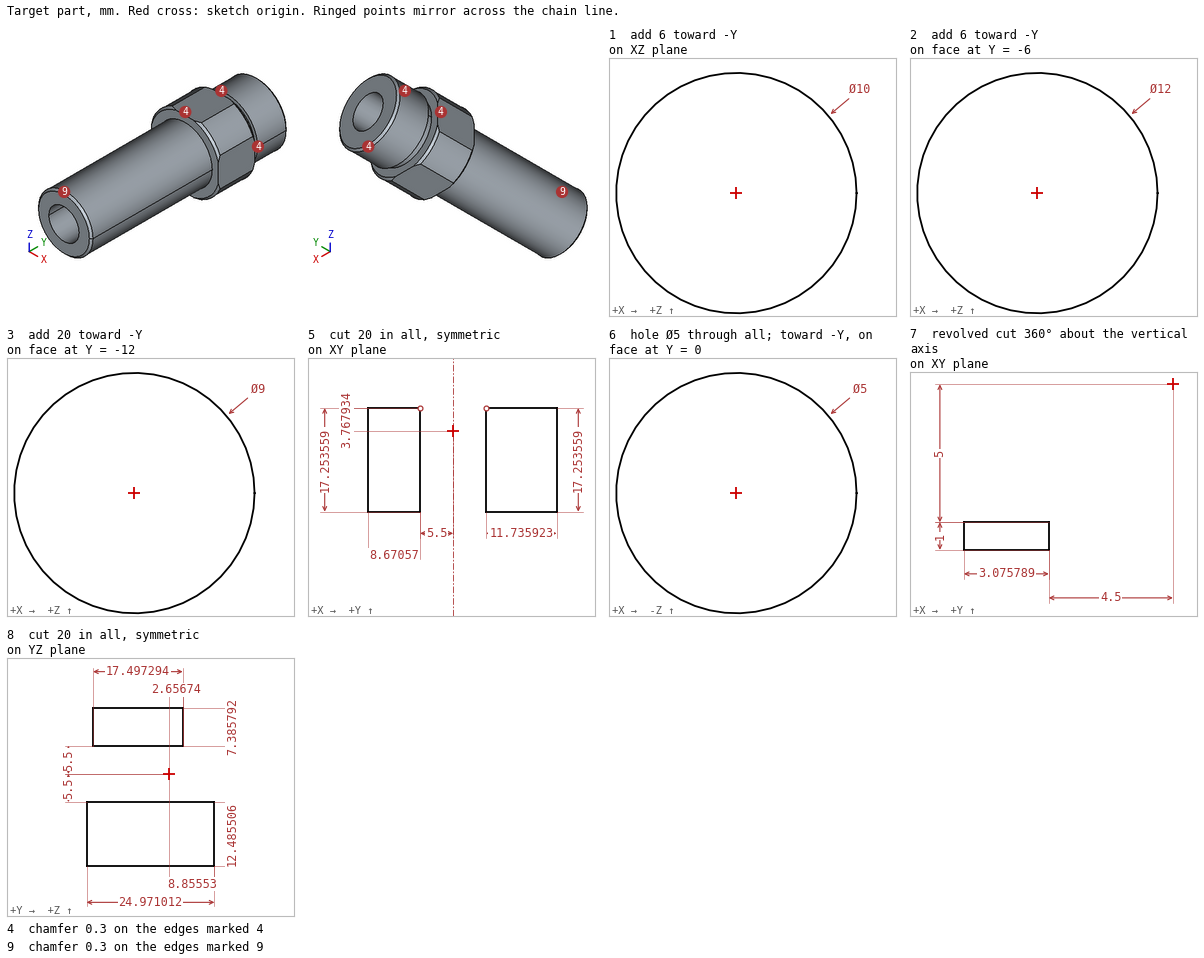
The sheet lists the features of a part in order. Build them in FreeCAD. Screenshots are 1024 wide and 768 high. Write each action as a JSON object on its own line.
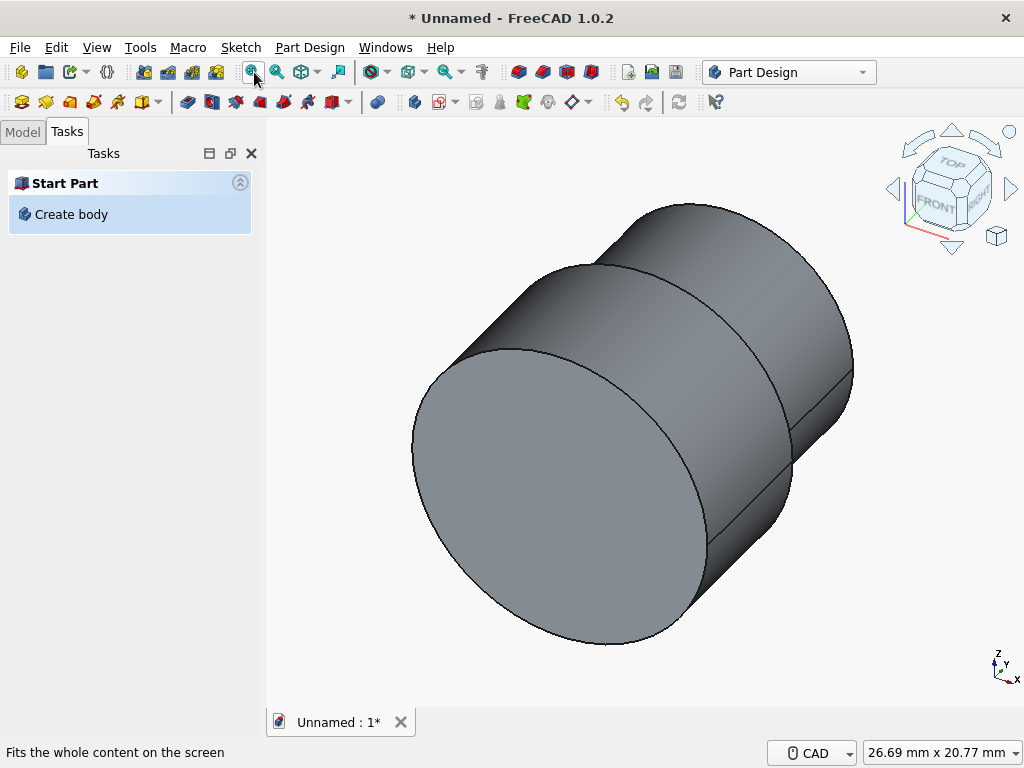
{"action": "left_click", "coordinate": [560, 496]}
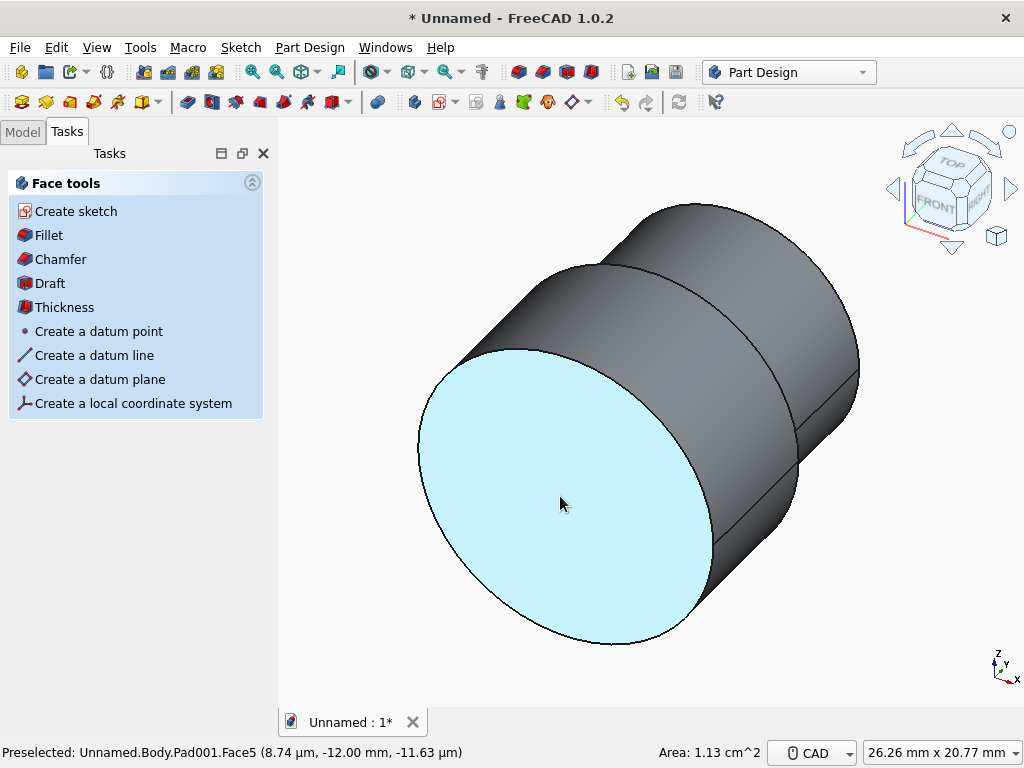
{"action": "left_click", "coordinate": [440, 102]}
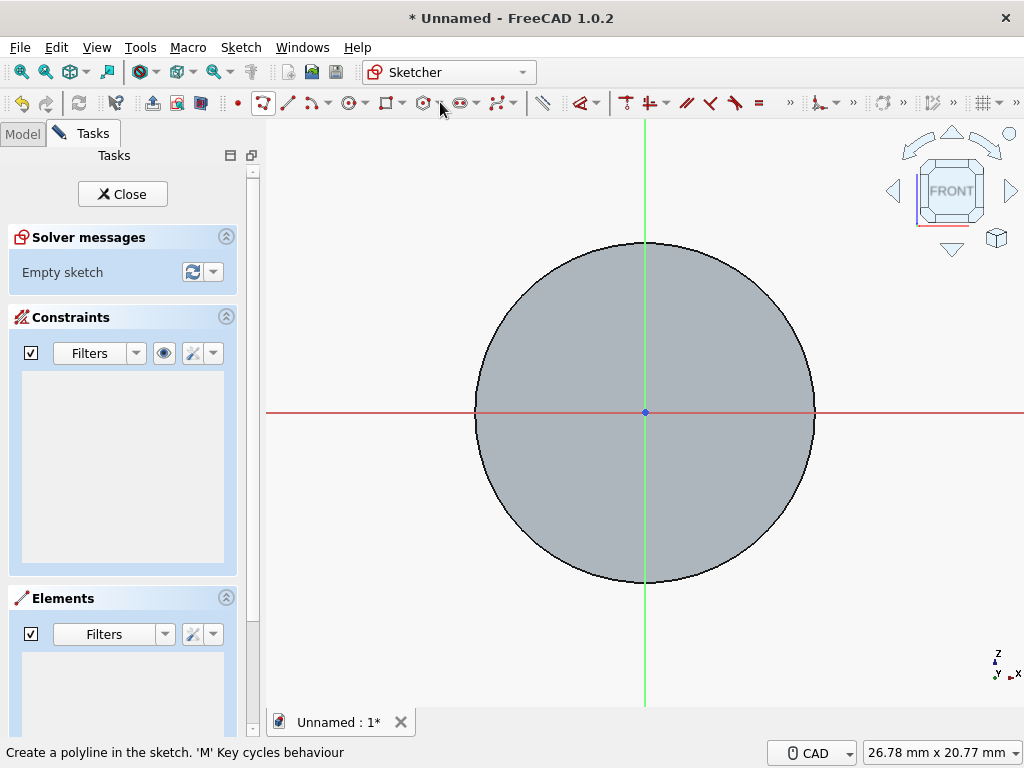
{"action": "scroll", "coordinate": [784, 413], "scroll_direction": "up", "scroll_amount": 2}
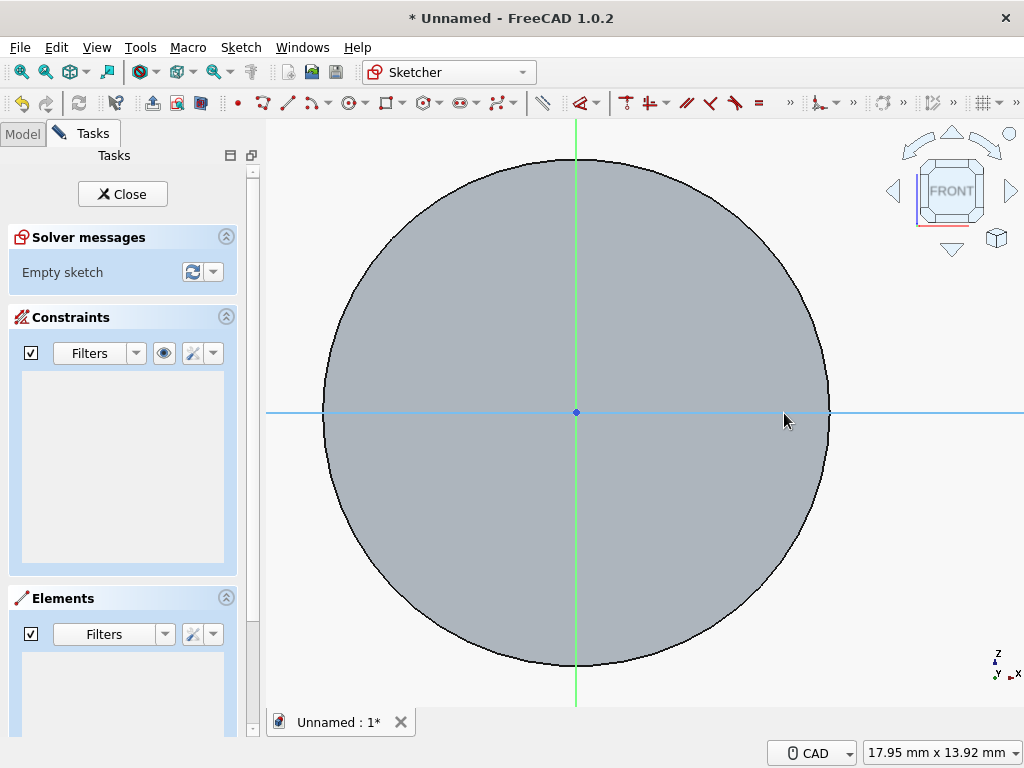
{"action": "key", "text": "g c"}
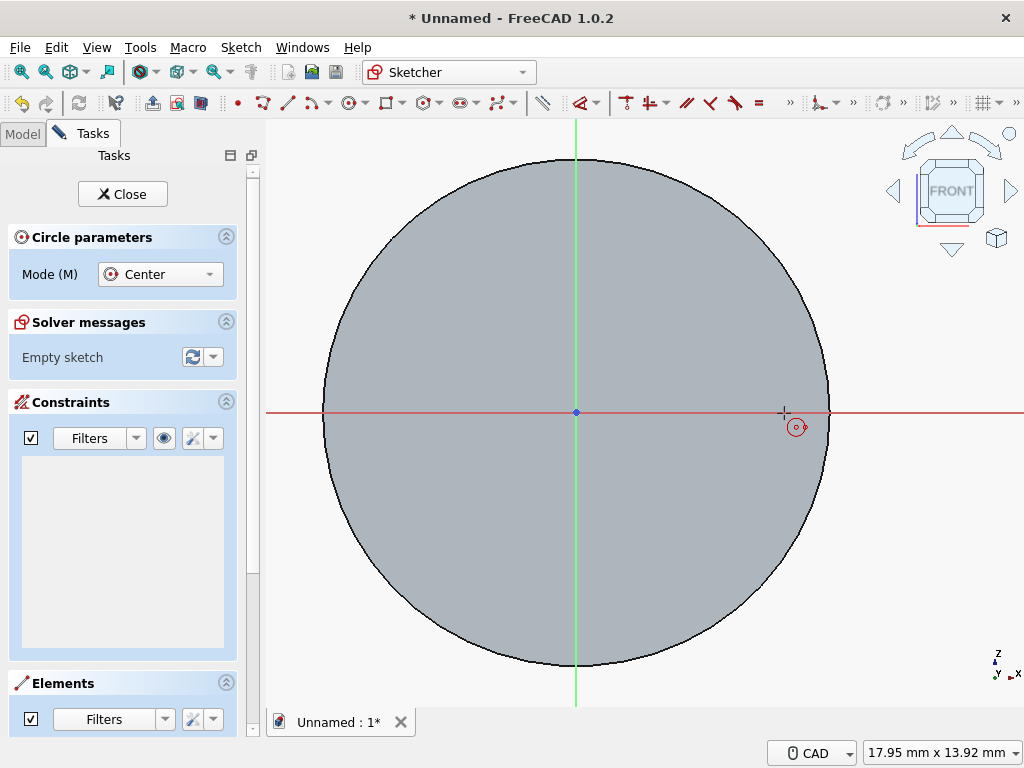
{"action": "left_click", "coordinate": [576, 413]}
{"action": "mouse_move", "coordinate": [711, 278]}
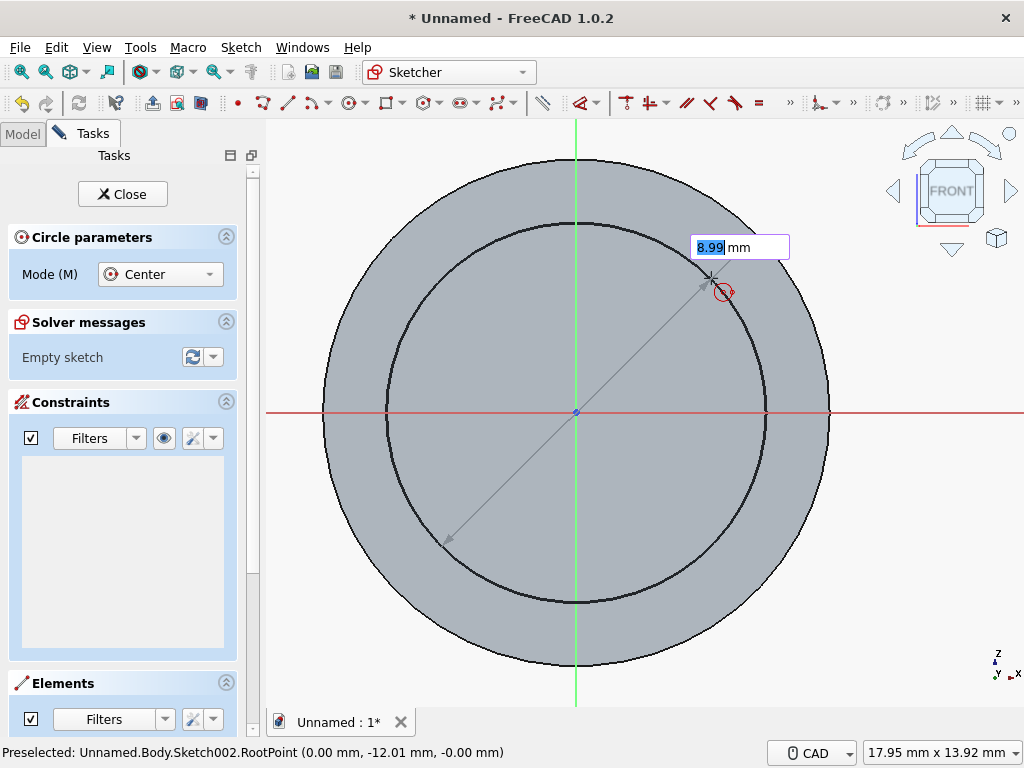
{"action": "type", "text": "9"}
{"action": "key", "text": "Return"}
{"action": "key", "text": "Escape"}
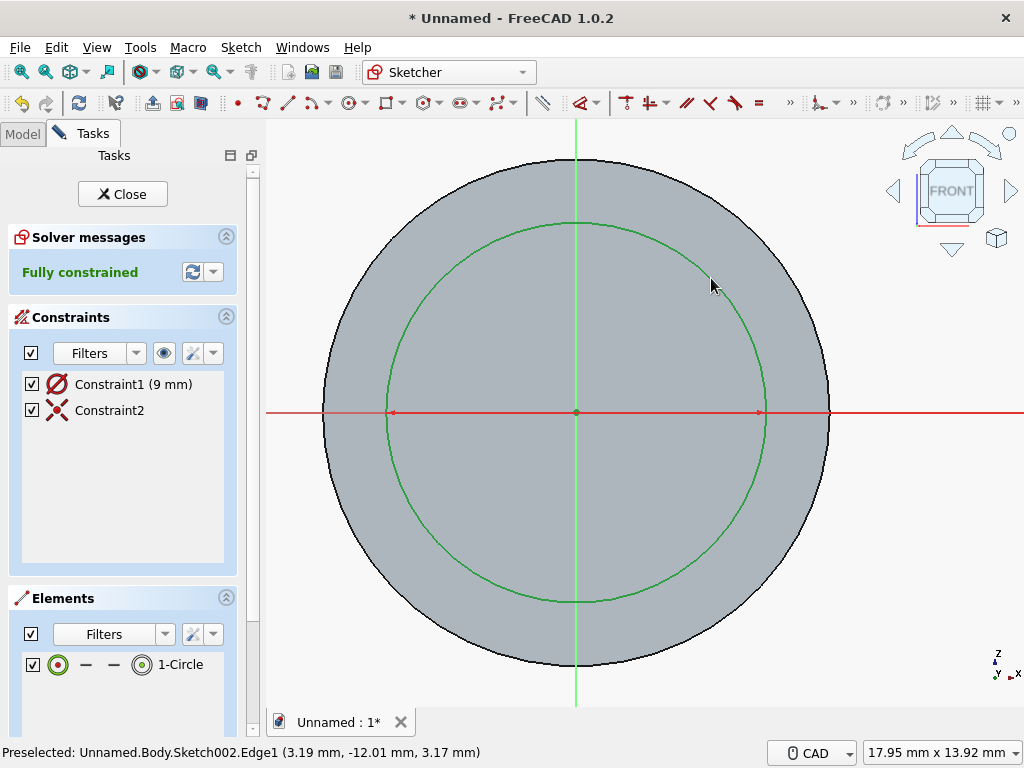
{"action": "left_click", "coordinate": [123, 194]}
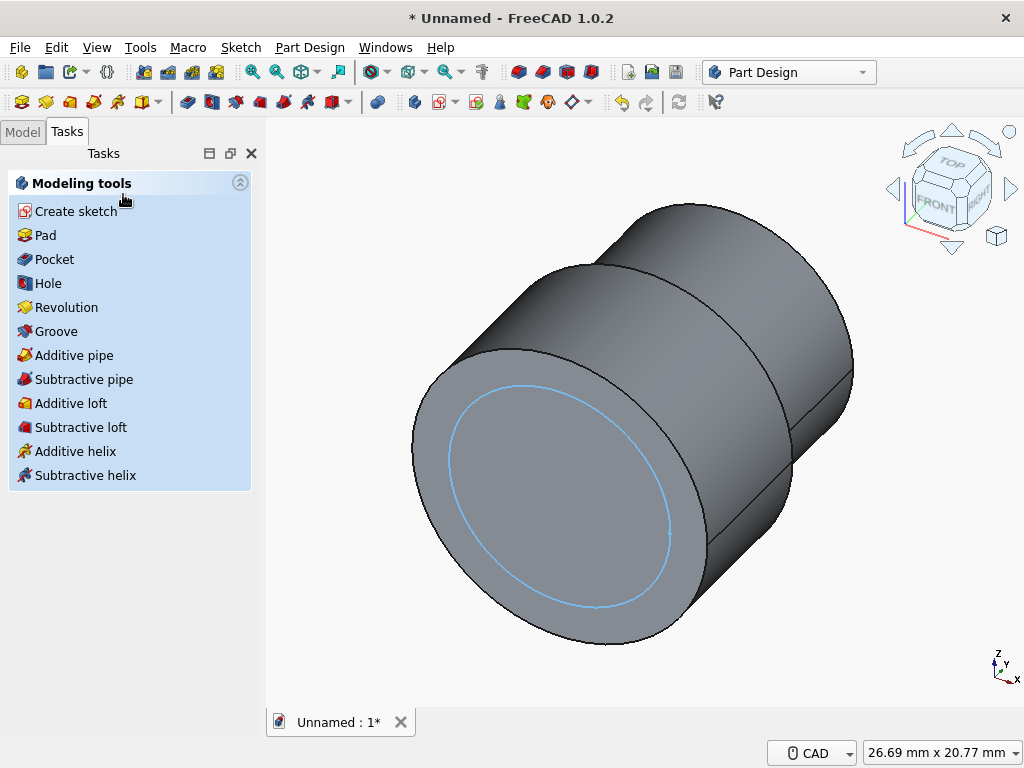
{"action": "left_click", "coordinate": [22, 102]}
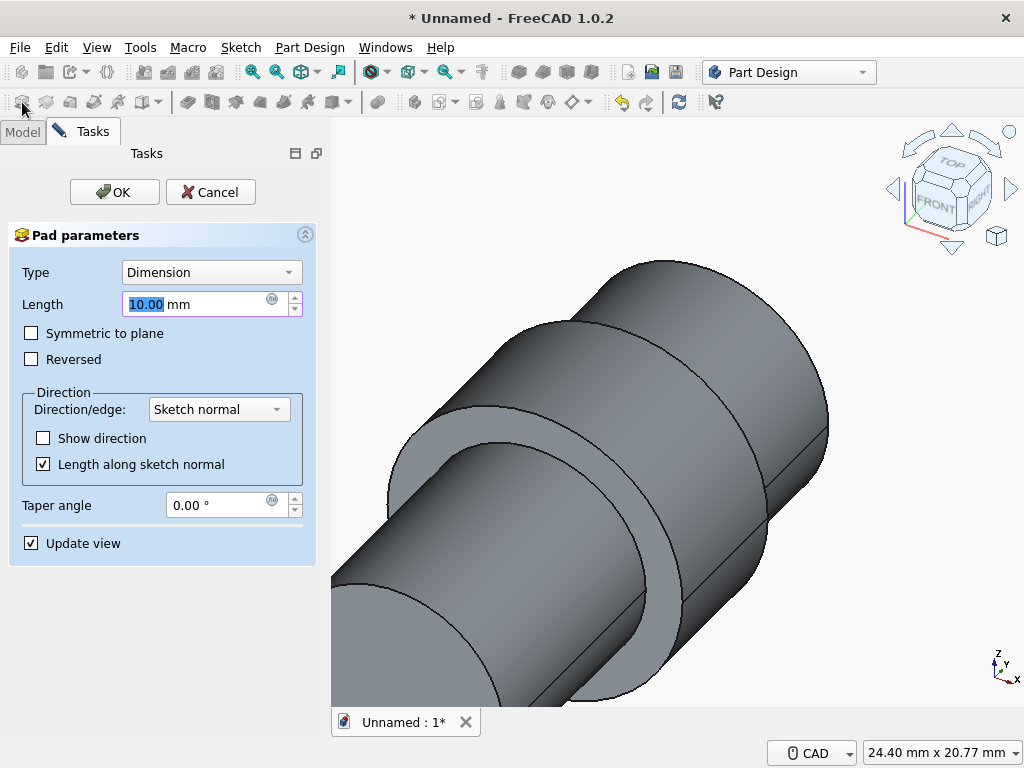
{"action": "type", "text": "20"}
{"action": "key", "text": "Tab"}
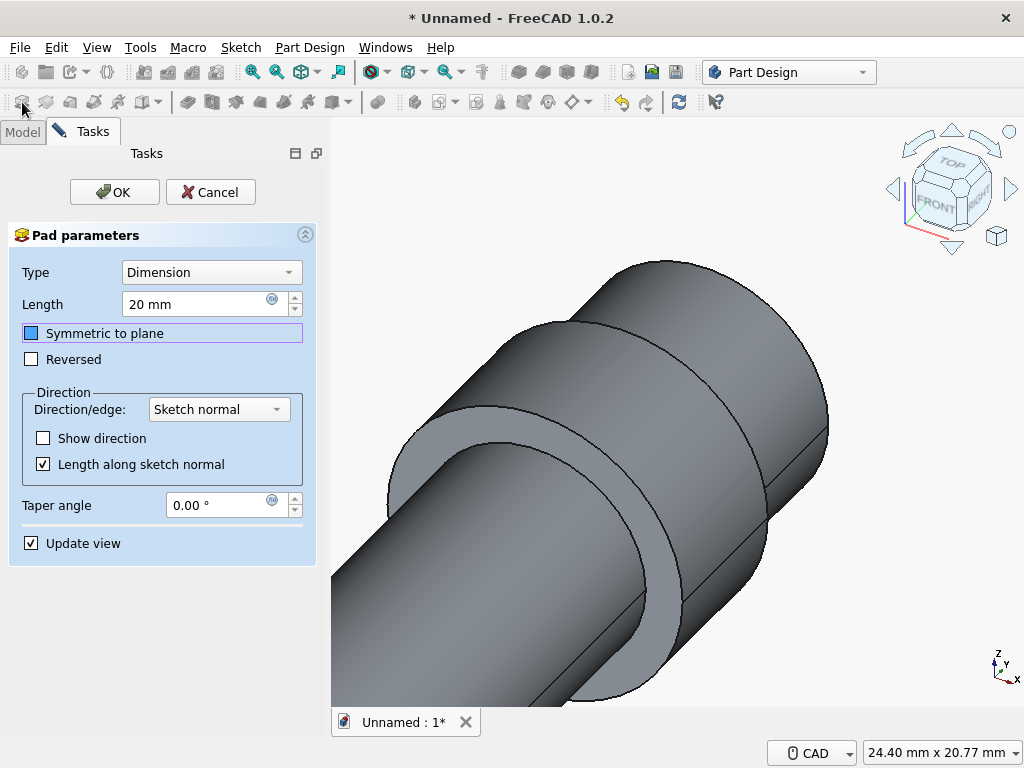
{"action": "left_click", "coordinate": [115, 192]}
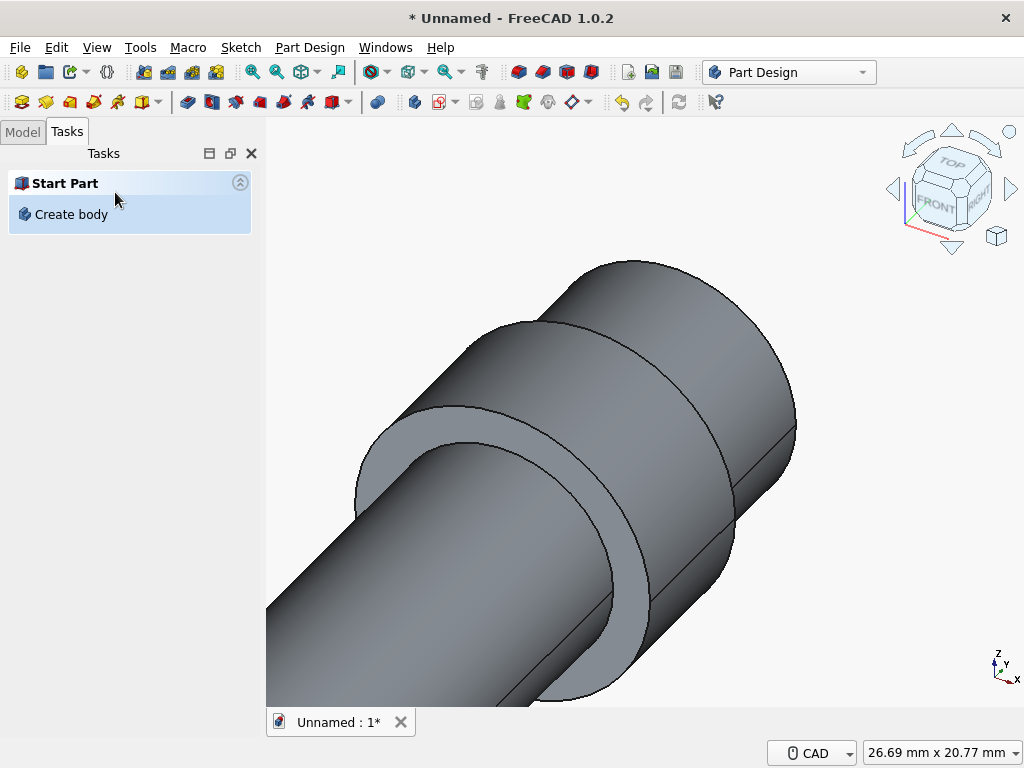
{"action": "key", "text": "v f"}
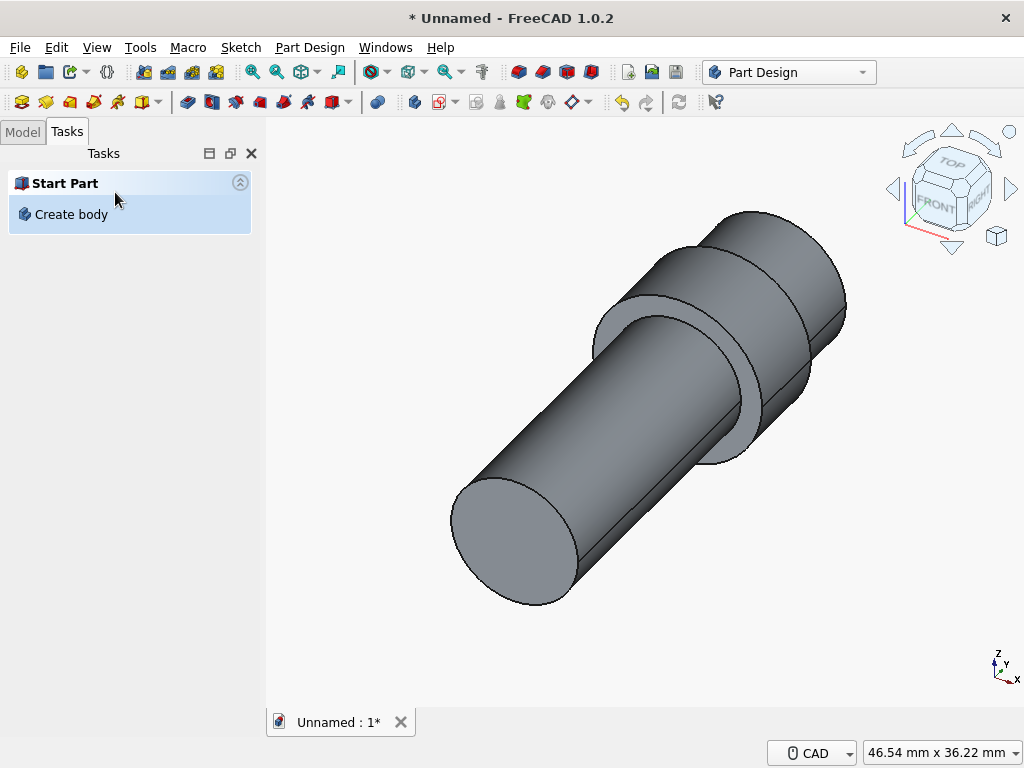
{"action": "left_click", "coordinate": [609, 309]}